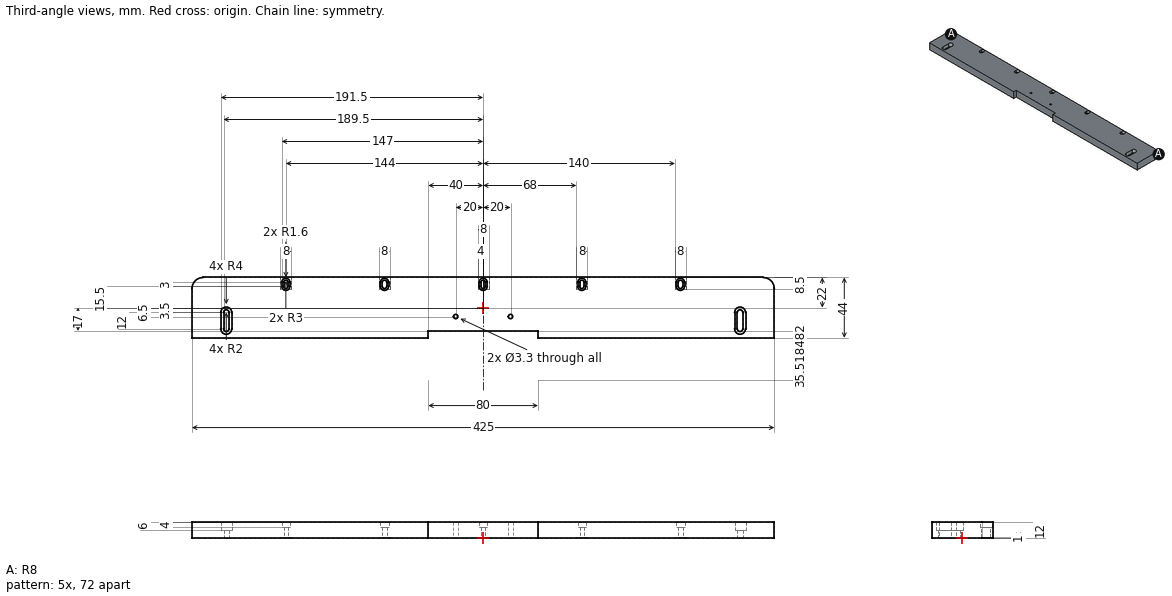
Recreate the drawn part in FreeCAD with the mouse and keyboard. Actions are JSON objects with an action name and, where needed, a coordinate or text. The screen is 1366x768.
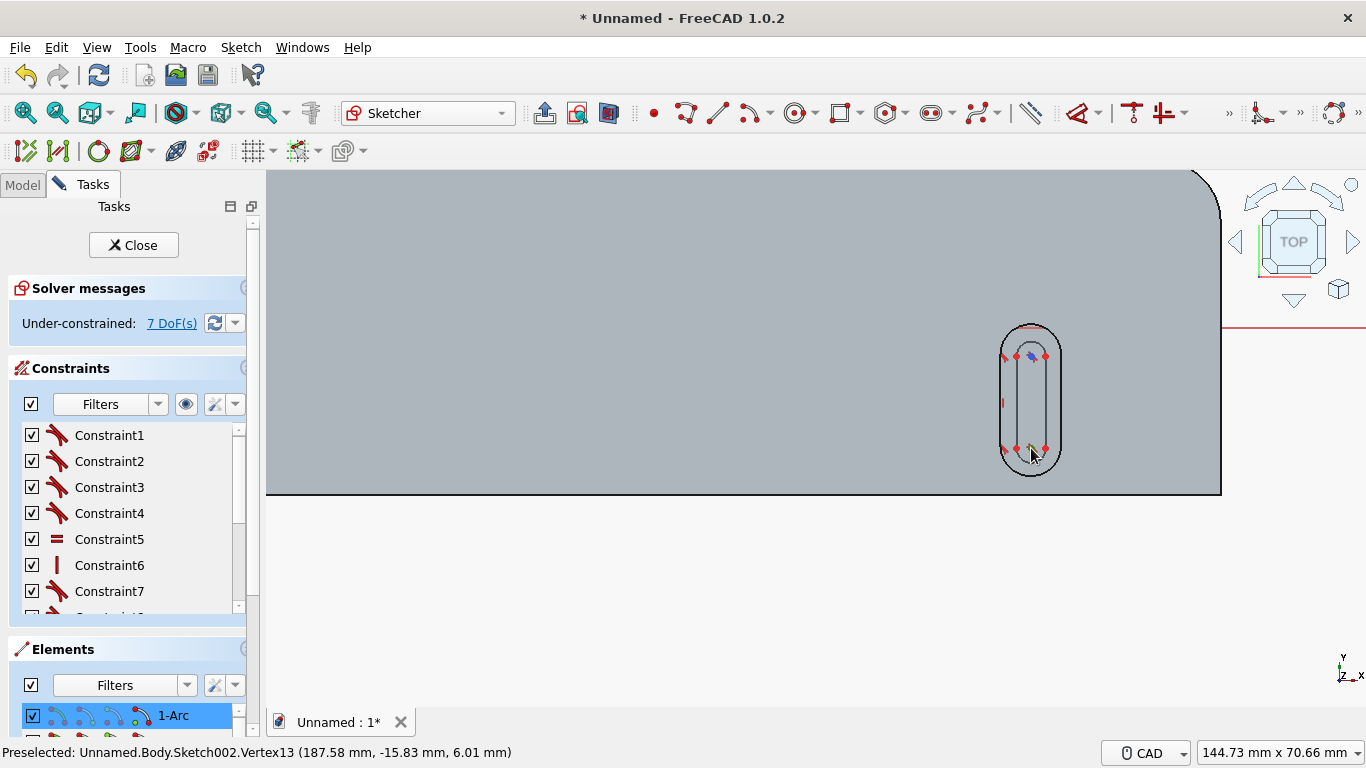
{"action": "scroll", "coordinate": [1036, 450], "scroll_direction": "down", "scroll_amount": 8}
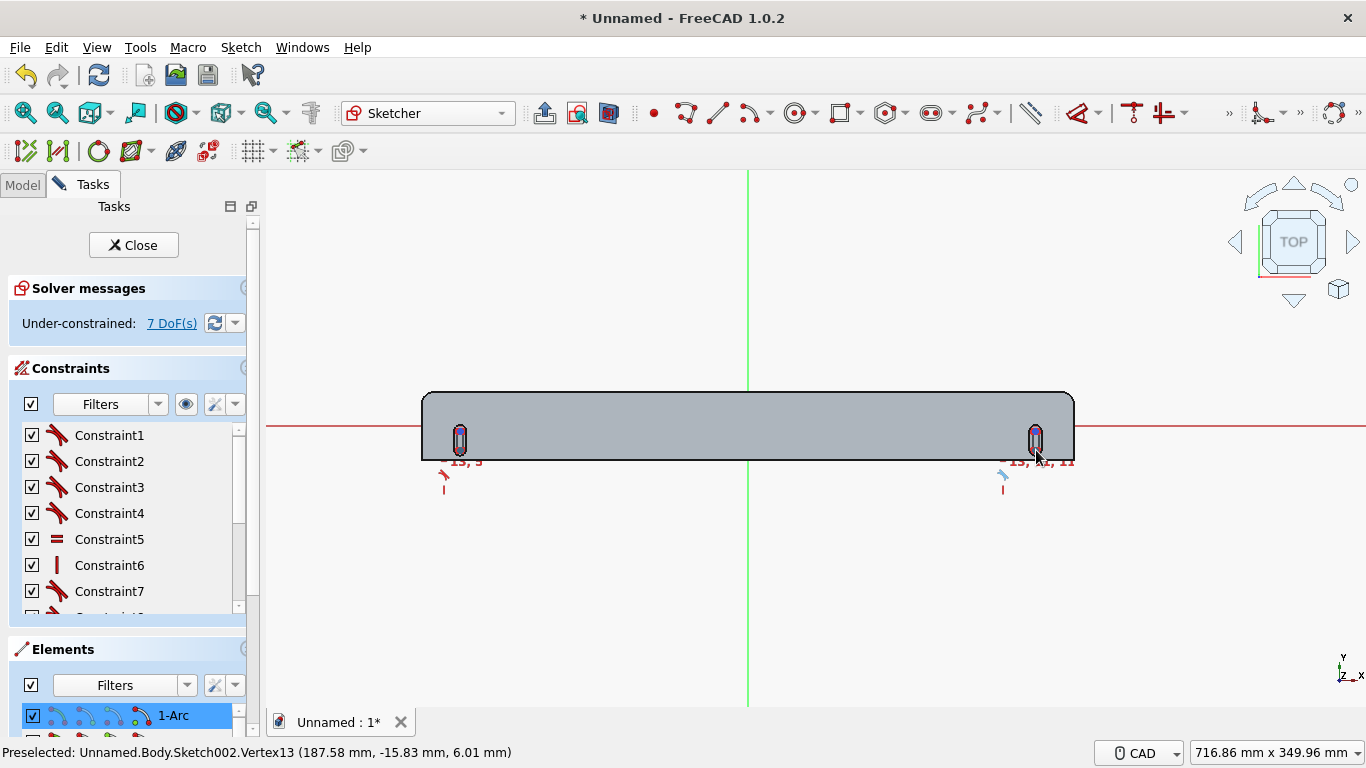
{"action": "left_click", "coordinate": [748, 645]}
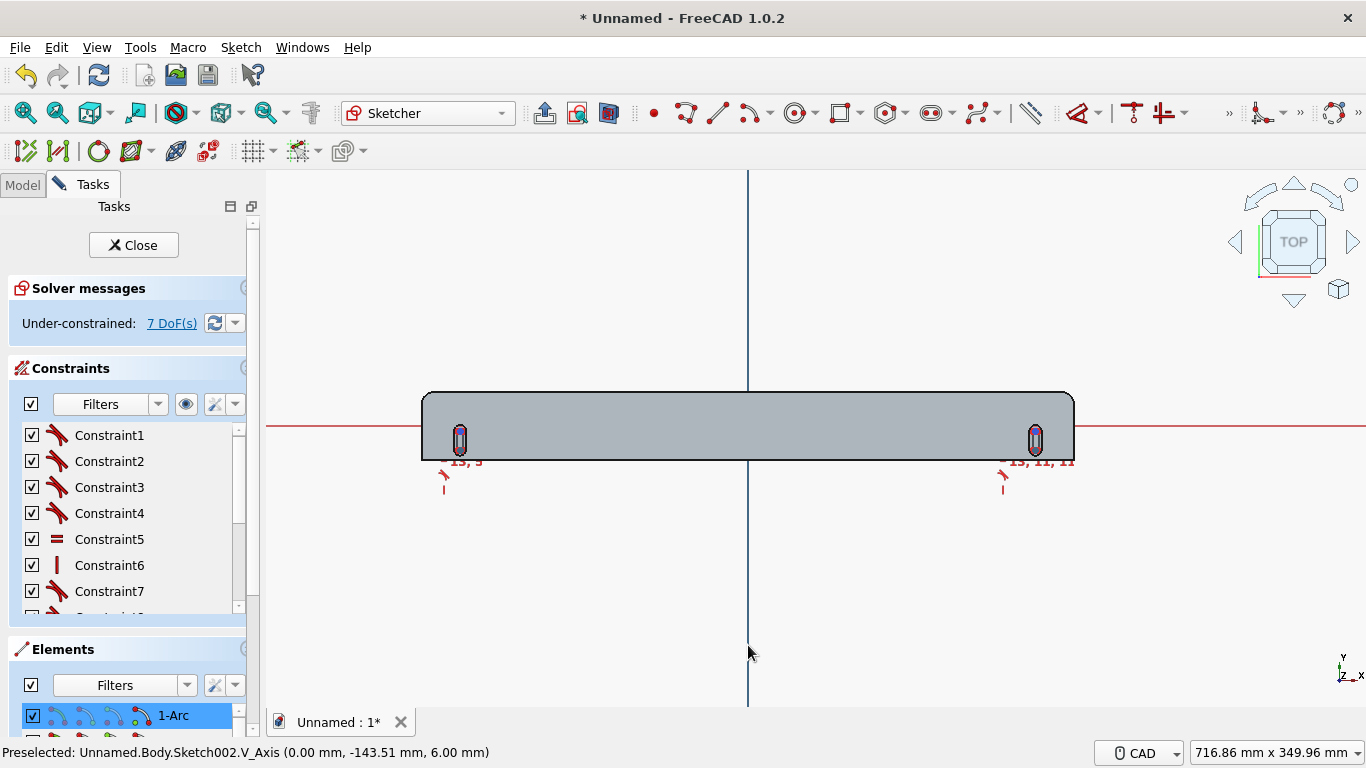
{"action": "key", "text": "s"}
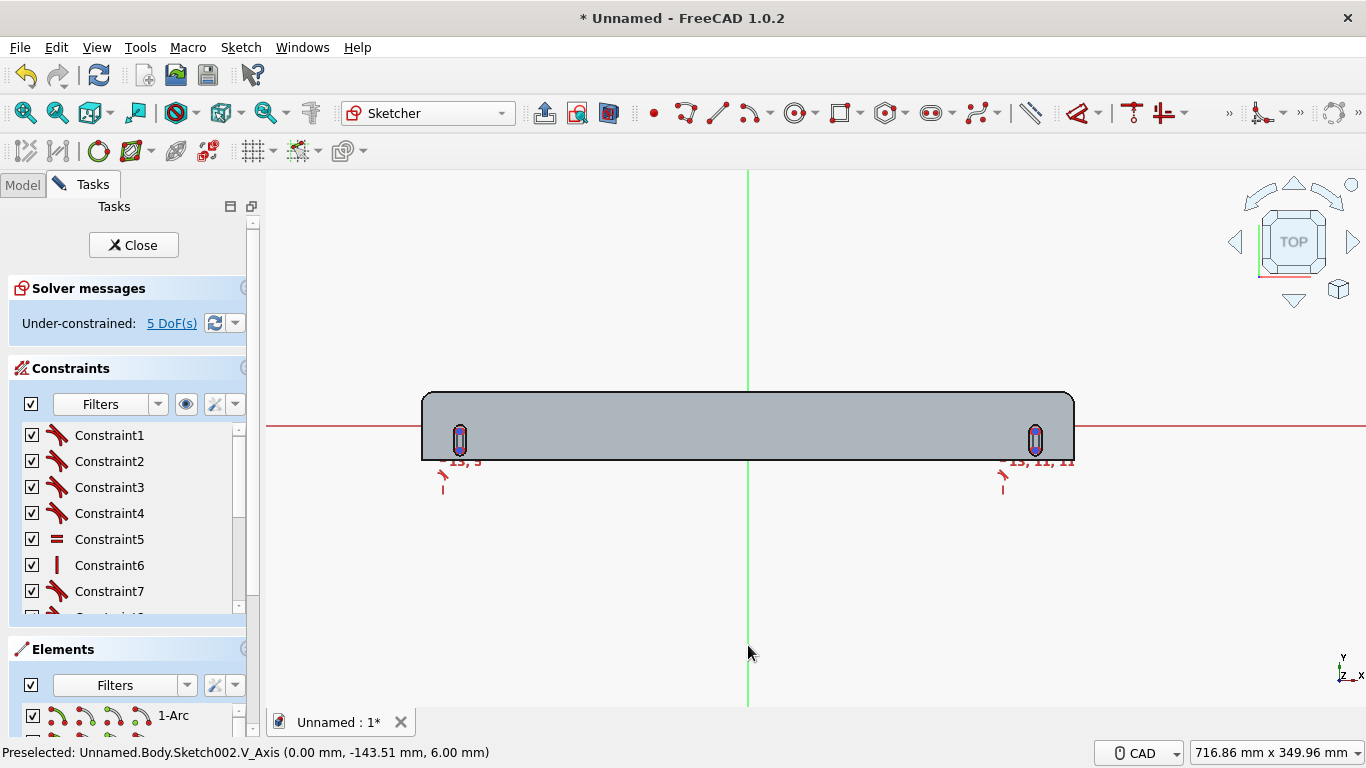
{"action": "left_click", "coordinate": [1078, 114]}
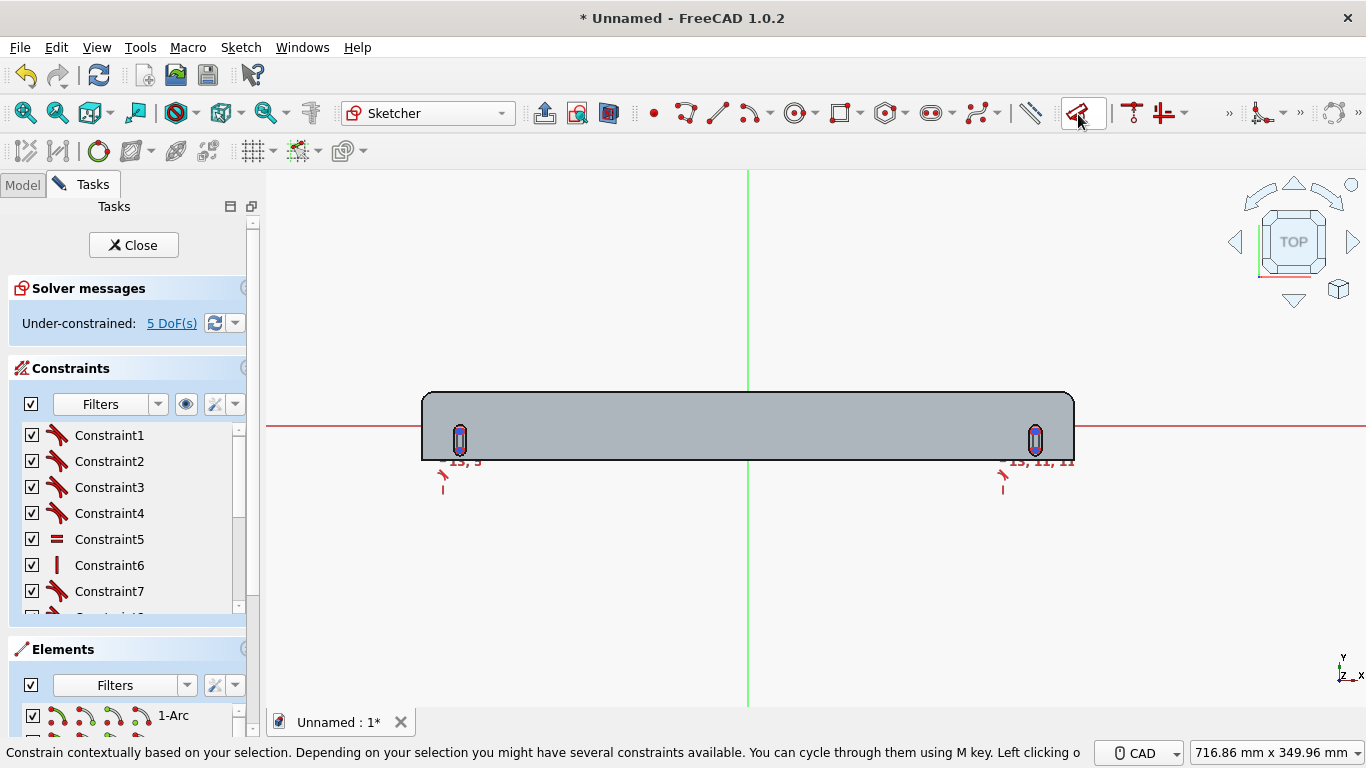
{"action": "scroll", "coordinate": [460, 453], "scroll_direction": "up", "scroll_amount": 13}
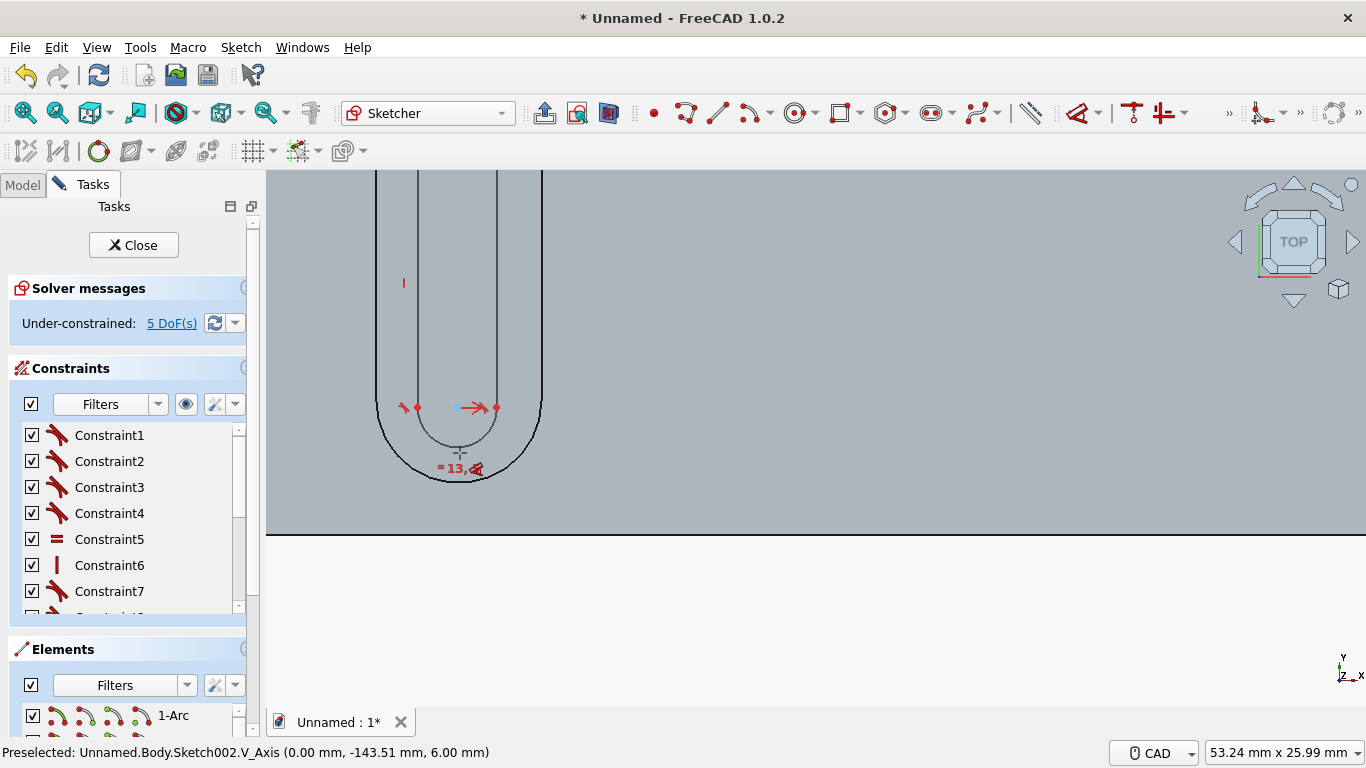
{"action": "left_click", "coordinate": [457, 447]}
{"action": "left_click", "coordinate": [457, 479]}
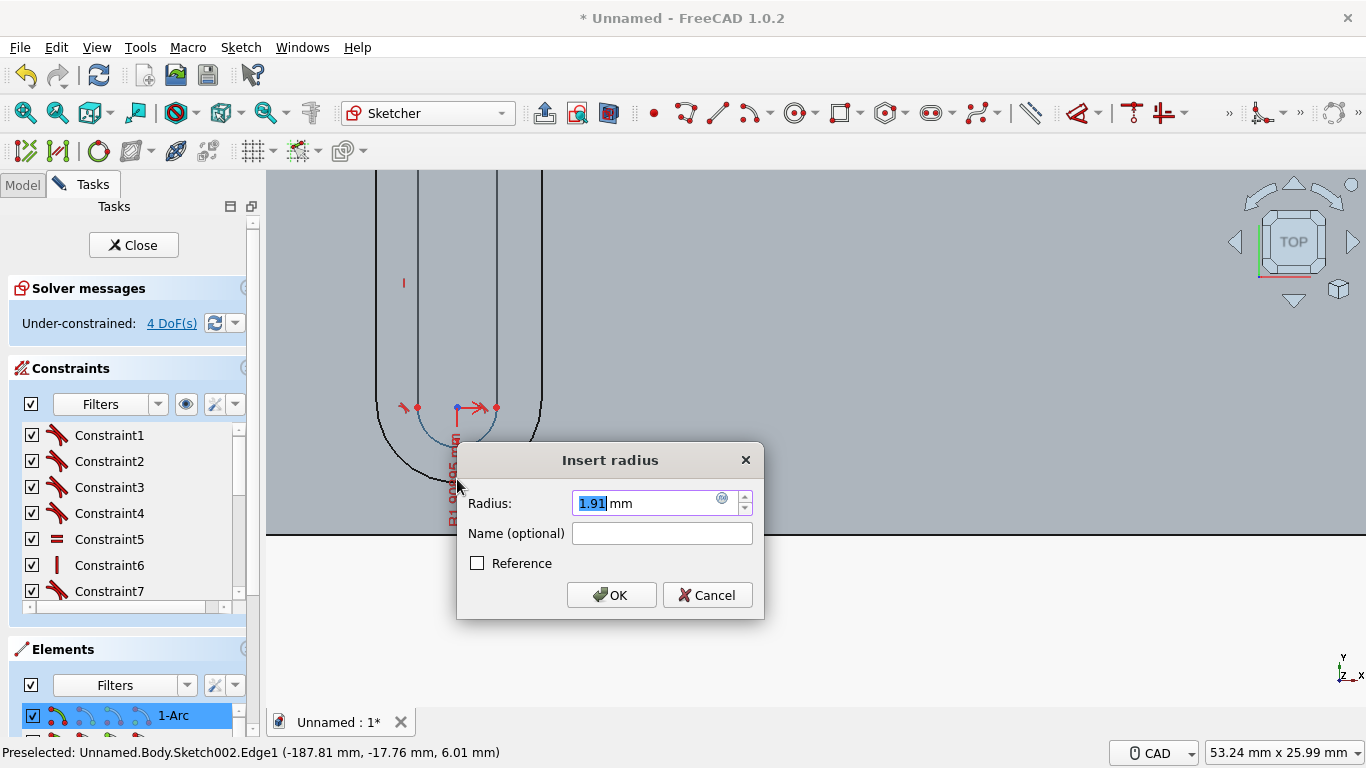
{"action": "type", "text": "2"}
{"action": "key", "text": "Return"}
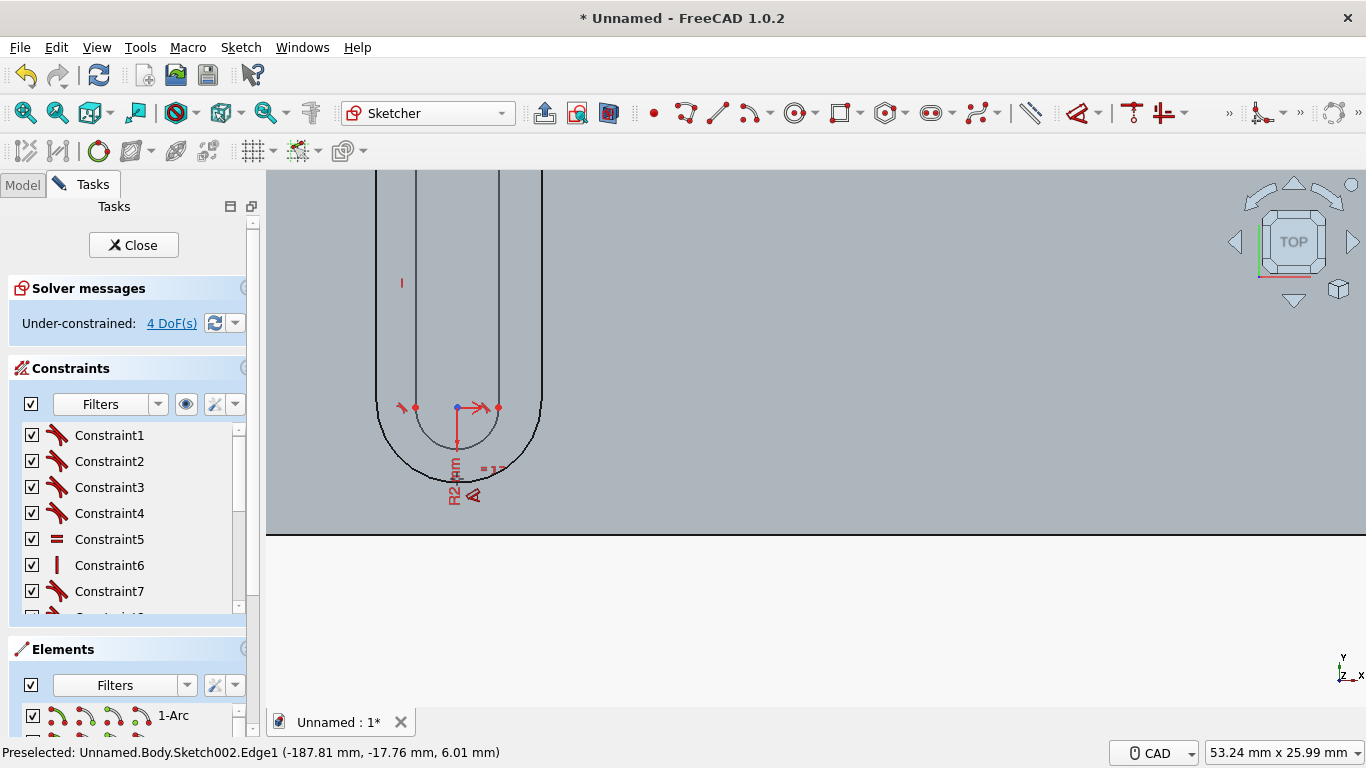
{"action": "scroll", "coordinate": [460, 453], "scroll_direction": "down", "scroll_amount": 13}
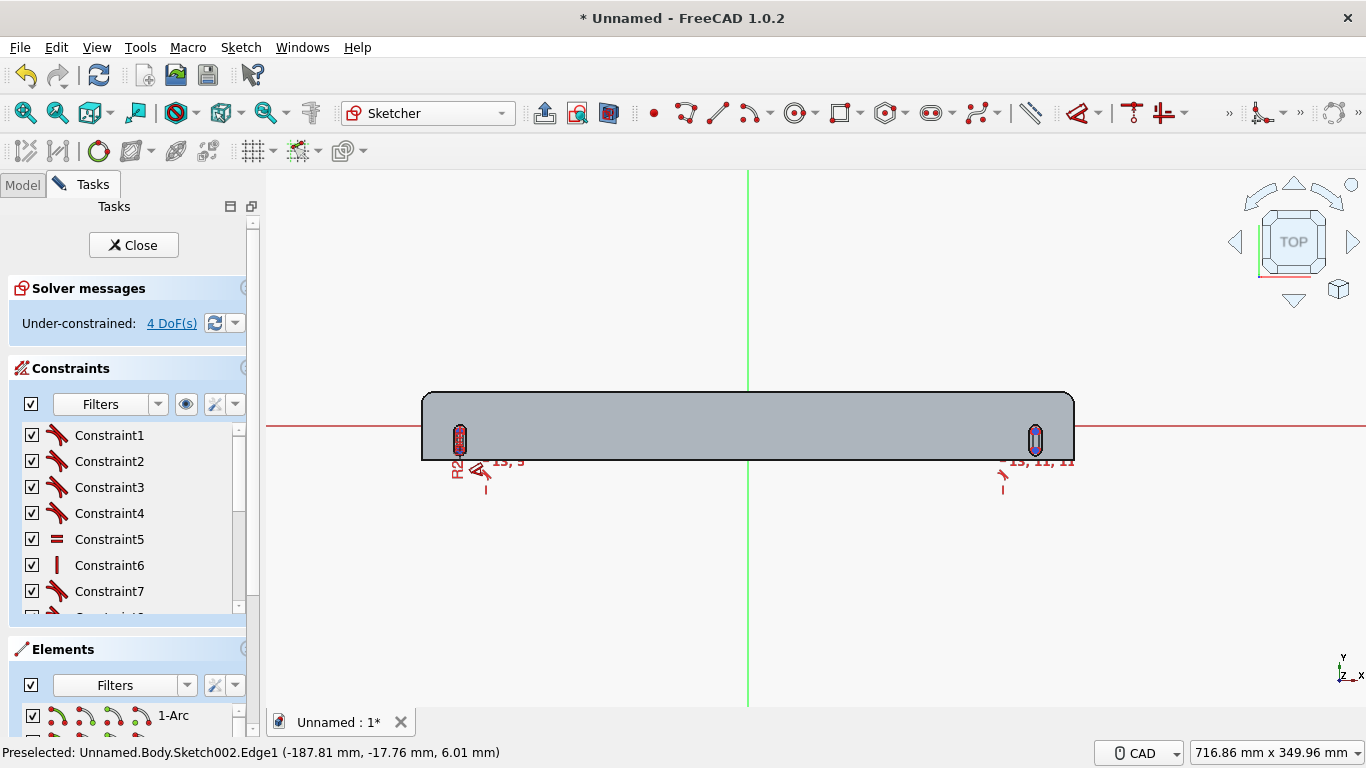
{"action": "scroll", "coordinate": [457, 445], "scroll_direction": "up", "scroll_amount": 5}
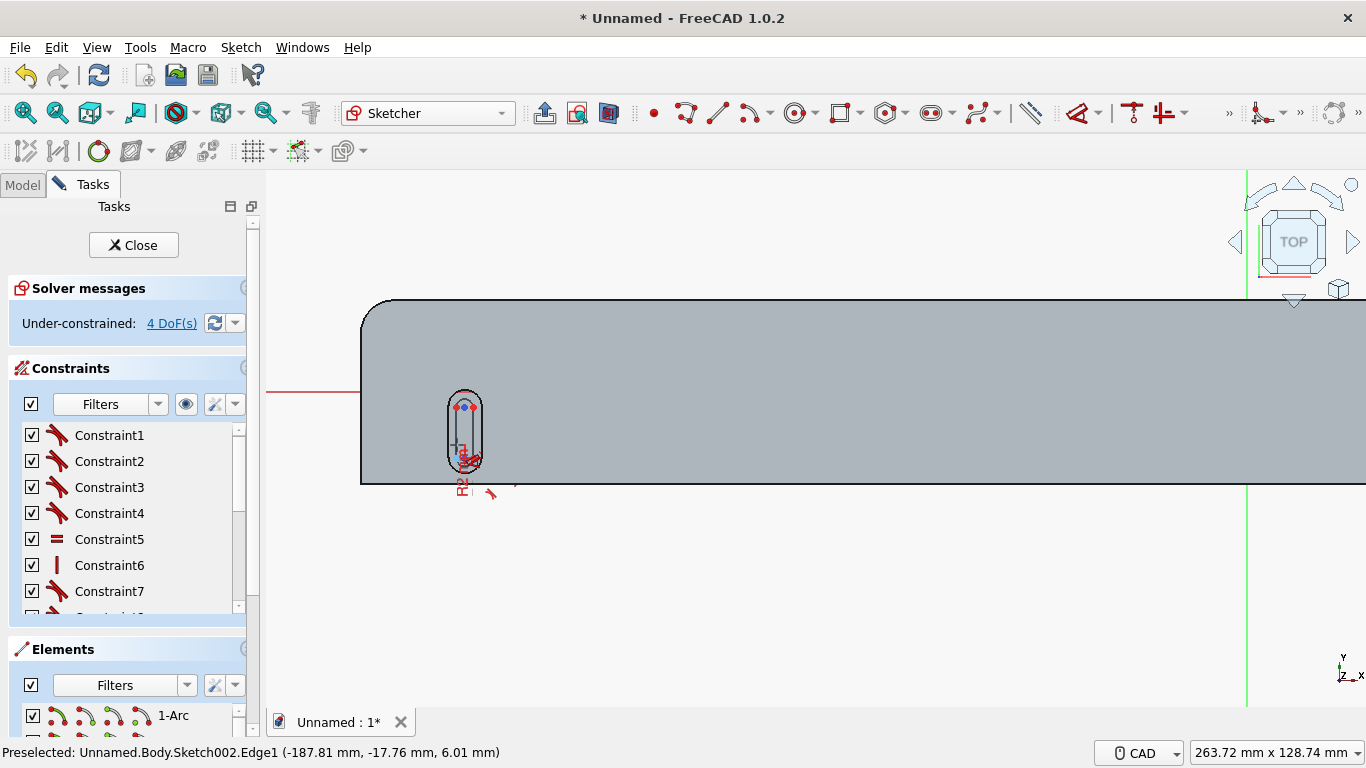
{"action": "left_click", "coordinate": [456, 443]}
{"action": "left_click", "coordinate": [422, 433]}